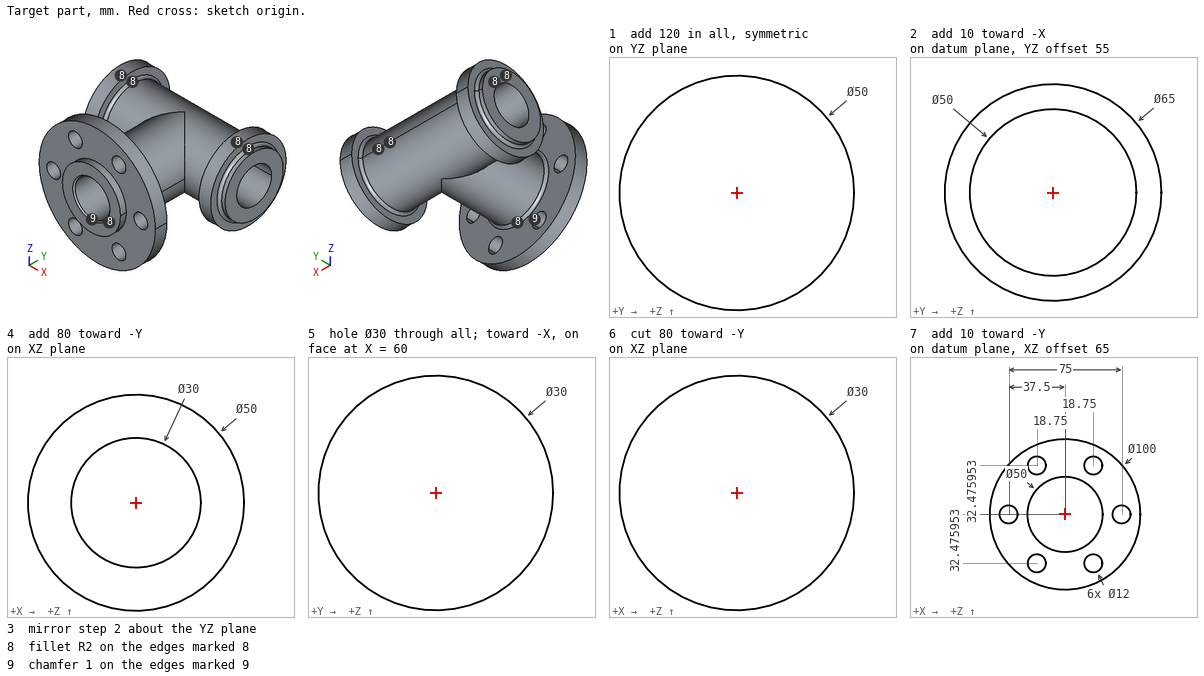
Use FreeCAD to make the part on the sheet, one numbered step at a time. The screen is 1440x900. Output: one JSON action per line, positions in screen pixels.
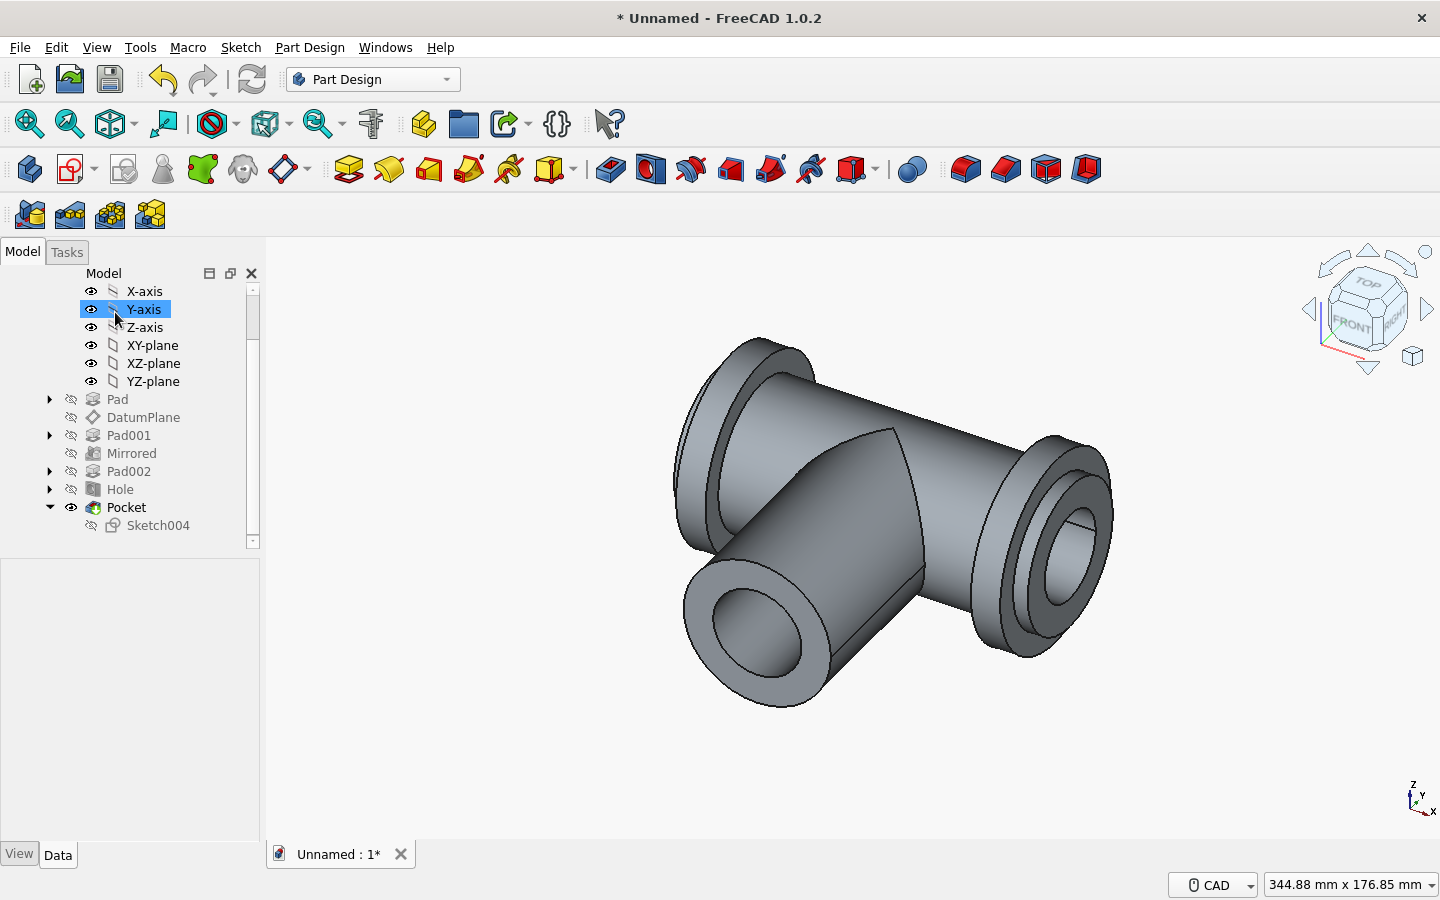
{"action": "scroll", "coordinate": [160, 413], "scroll_direction": "down", "scroll_amount": 3}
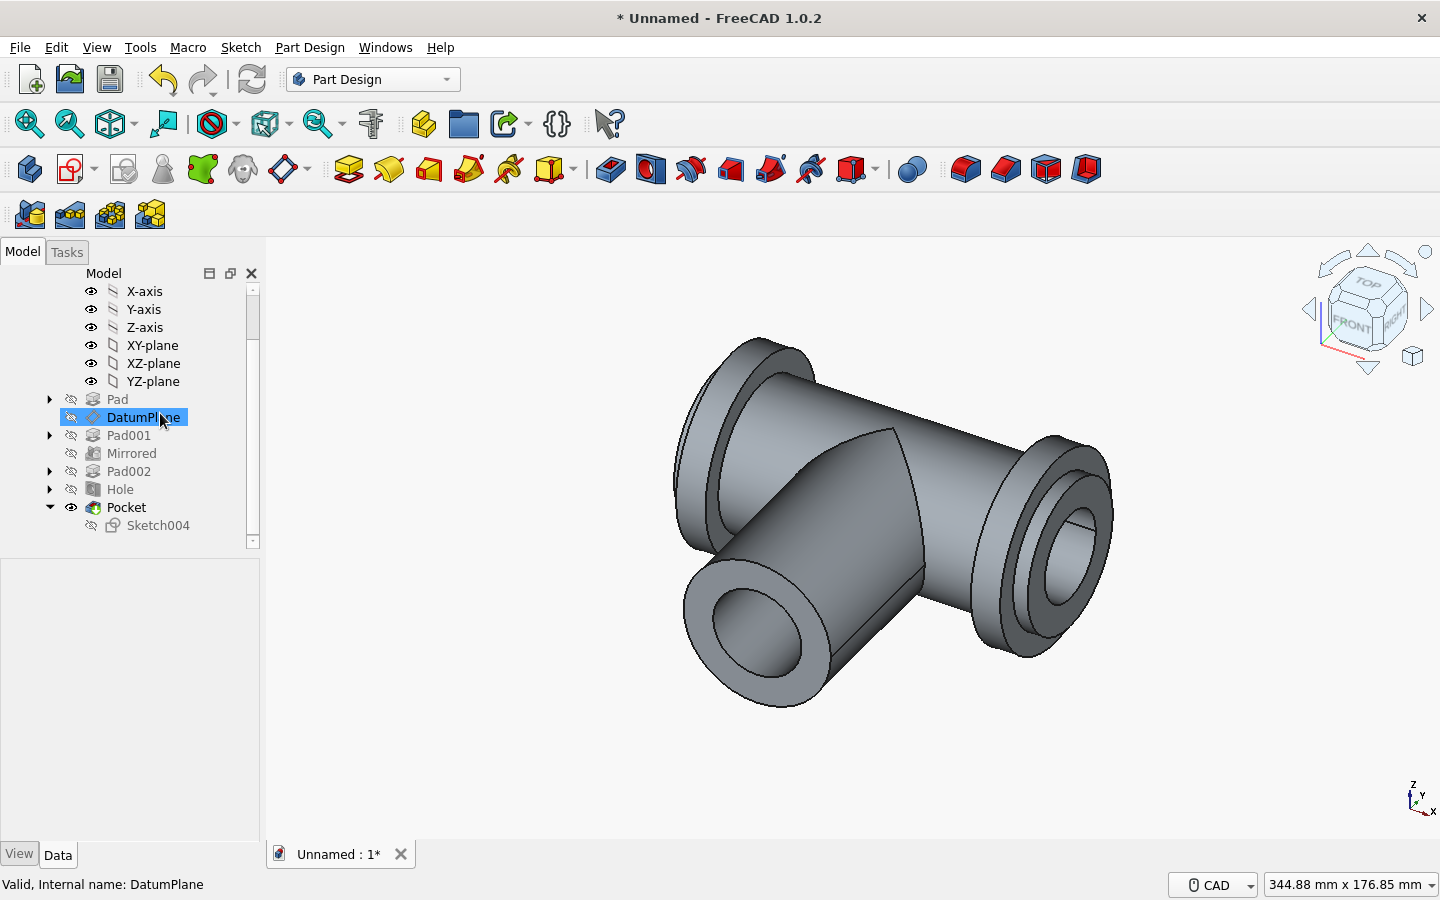
{"action": "scroll", "coordinate": [160, 413], "scroll_direction": "up", "scroll_amount": 15}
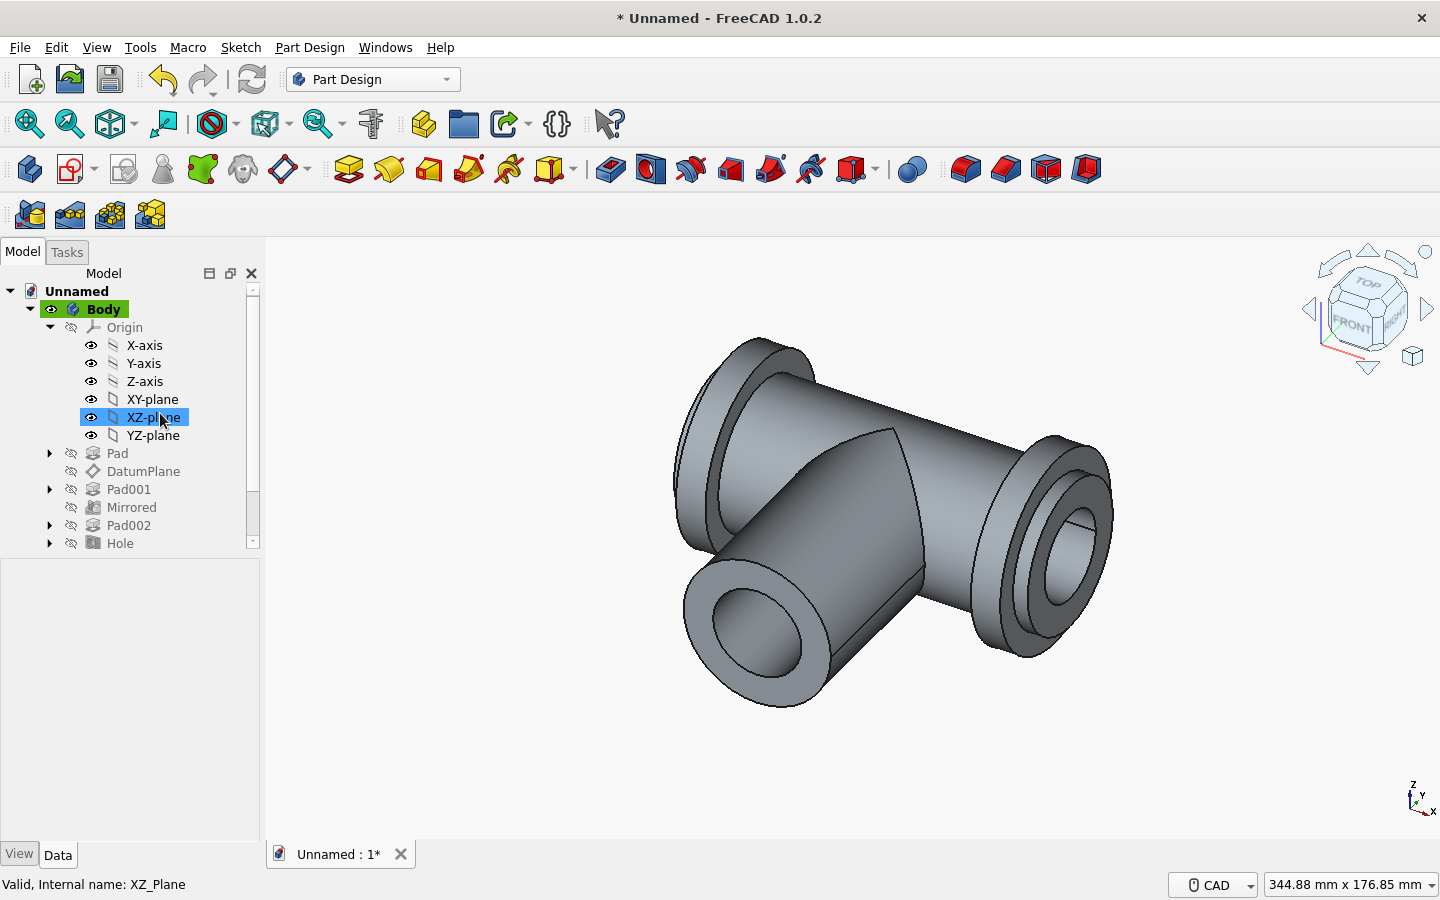
{"action": "left_click", "coordinate": [136, 417]}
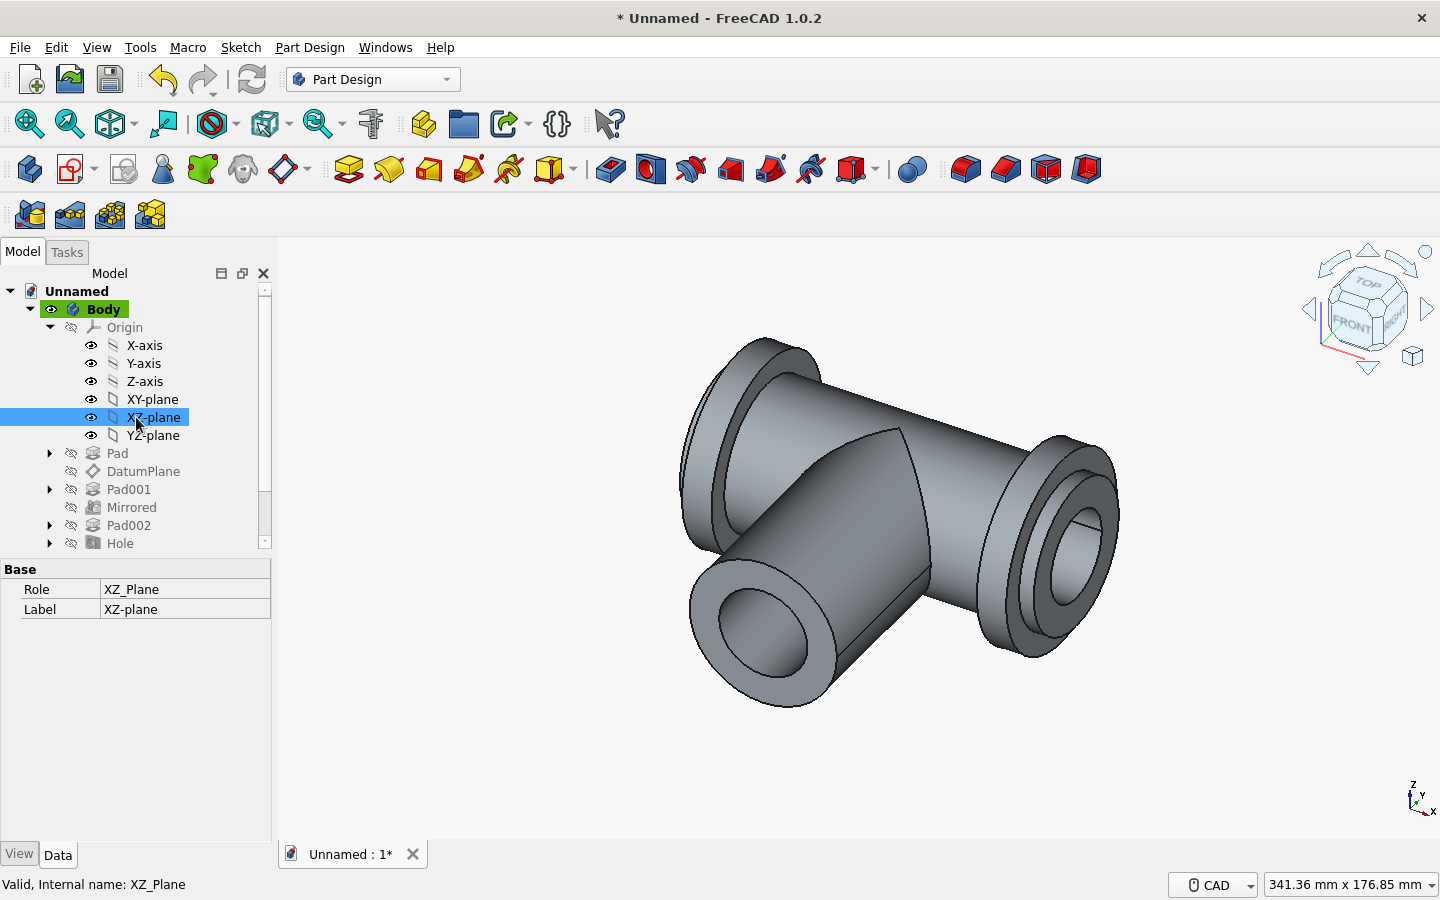
{"action": "left_click", "coordinate": [284, 170]}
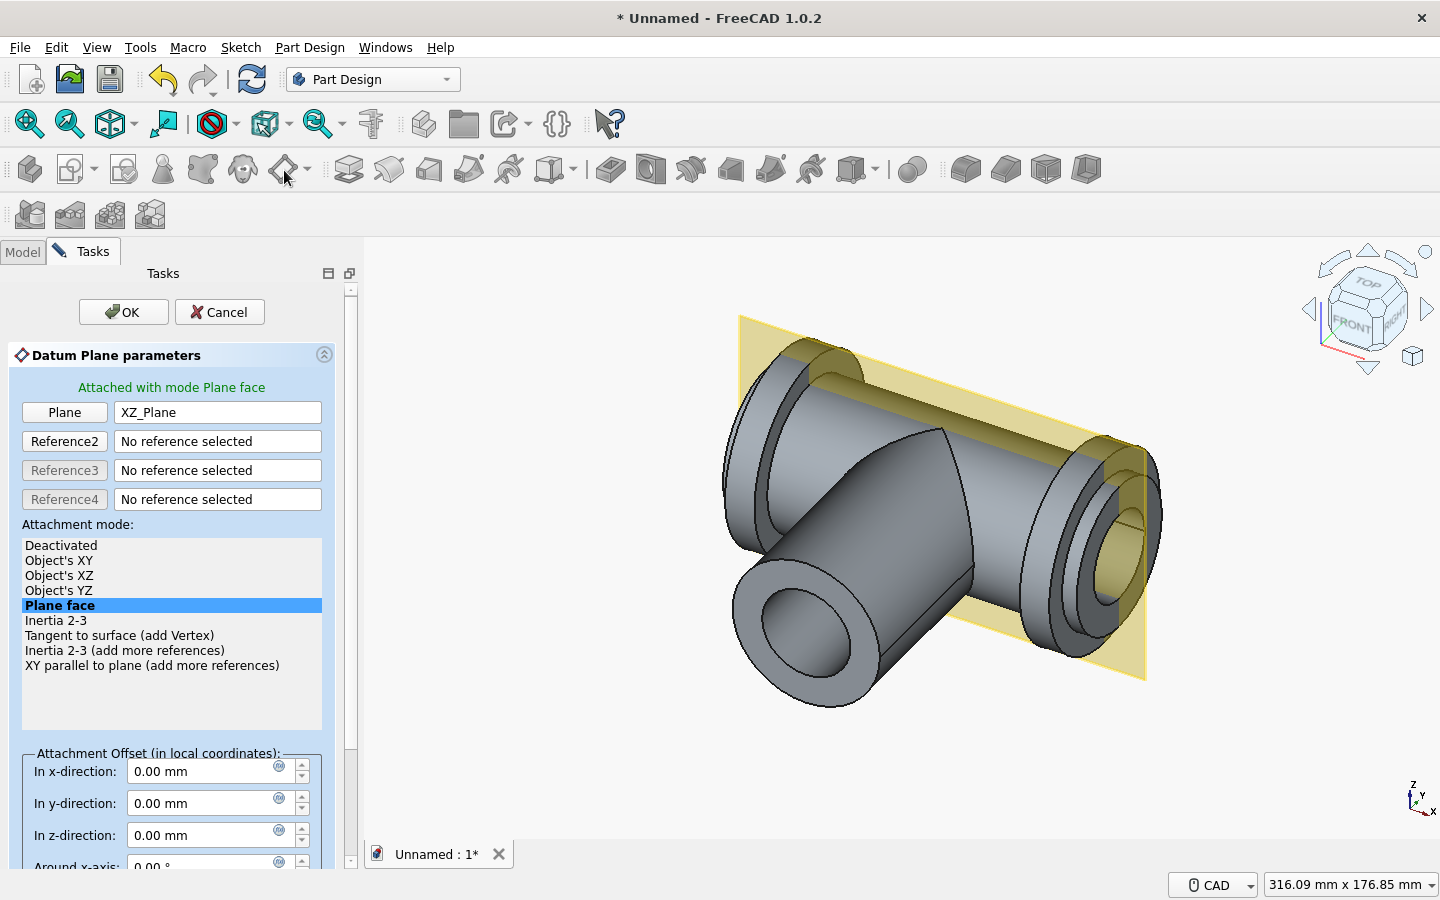
{"action": "triple_click", "coordinate": [210, 835]}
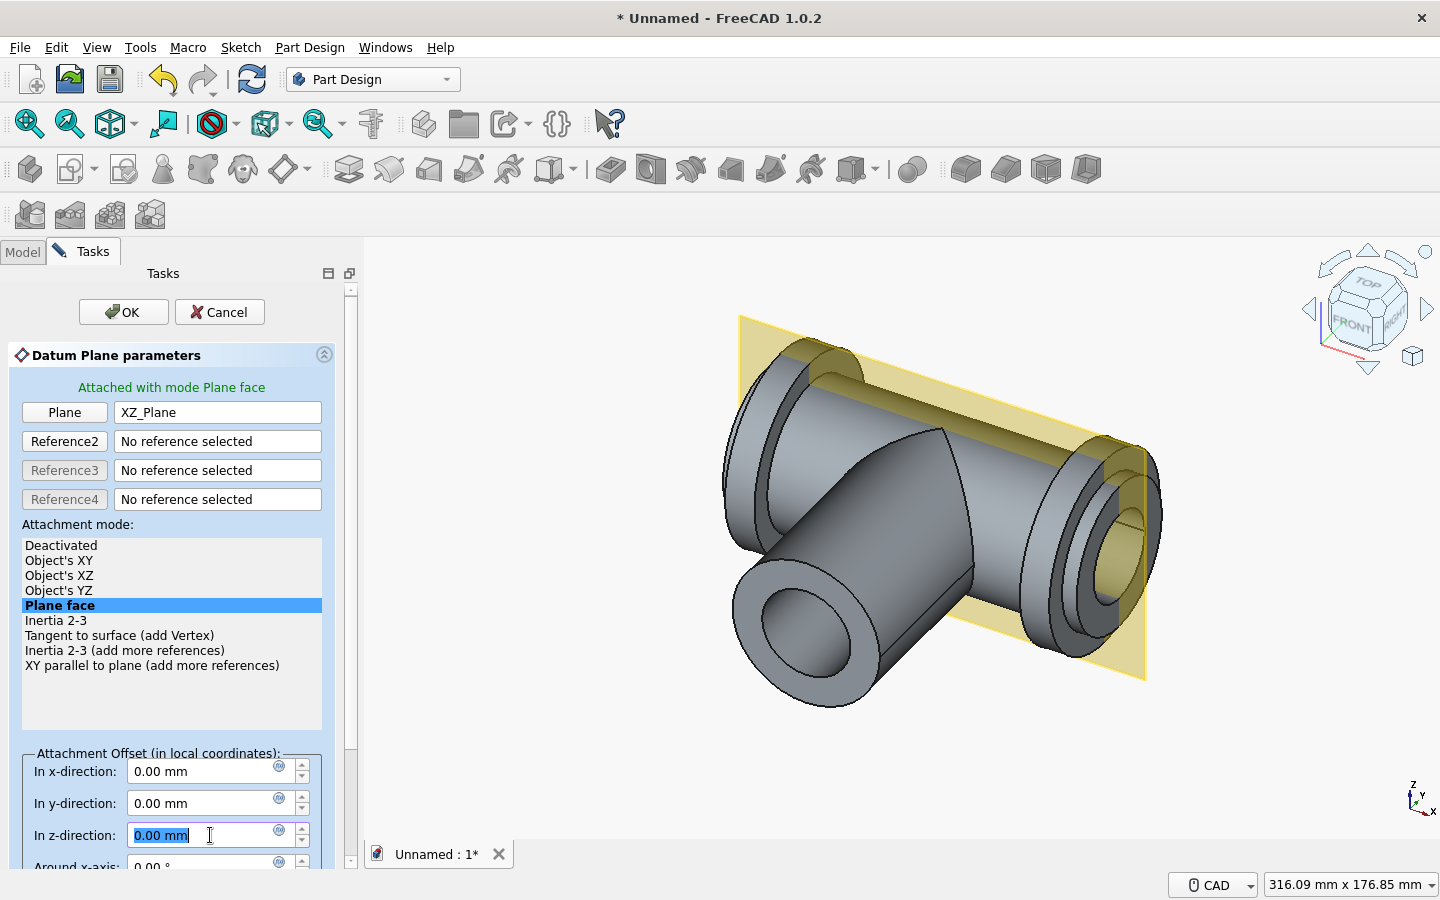
{"action": "type", "text": "65"}
{"action": "key", "text": "Tab"}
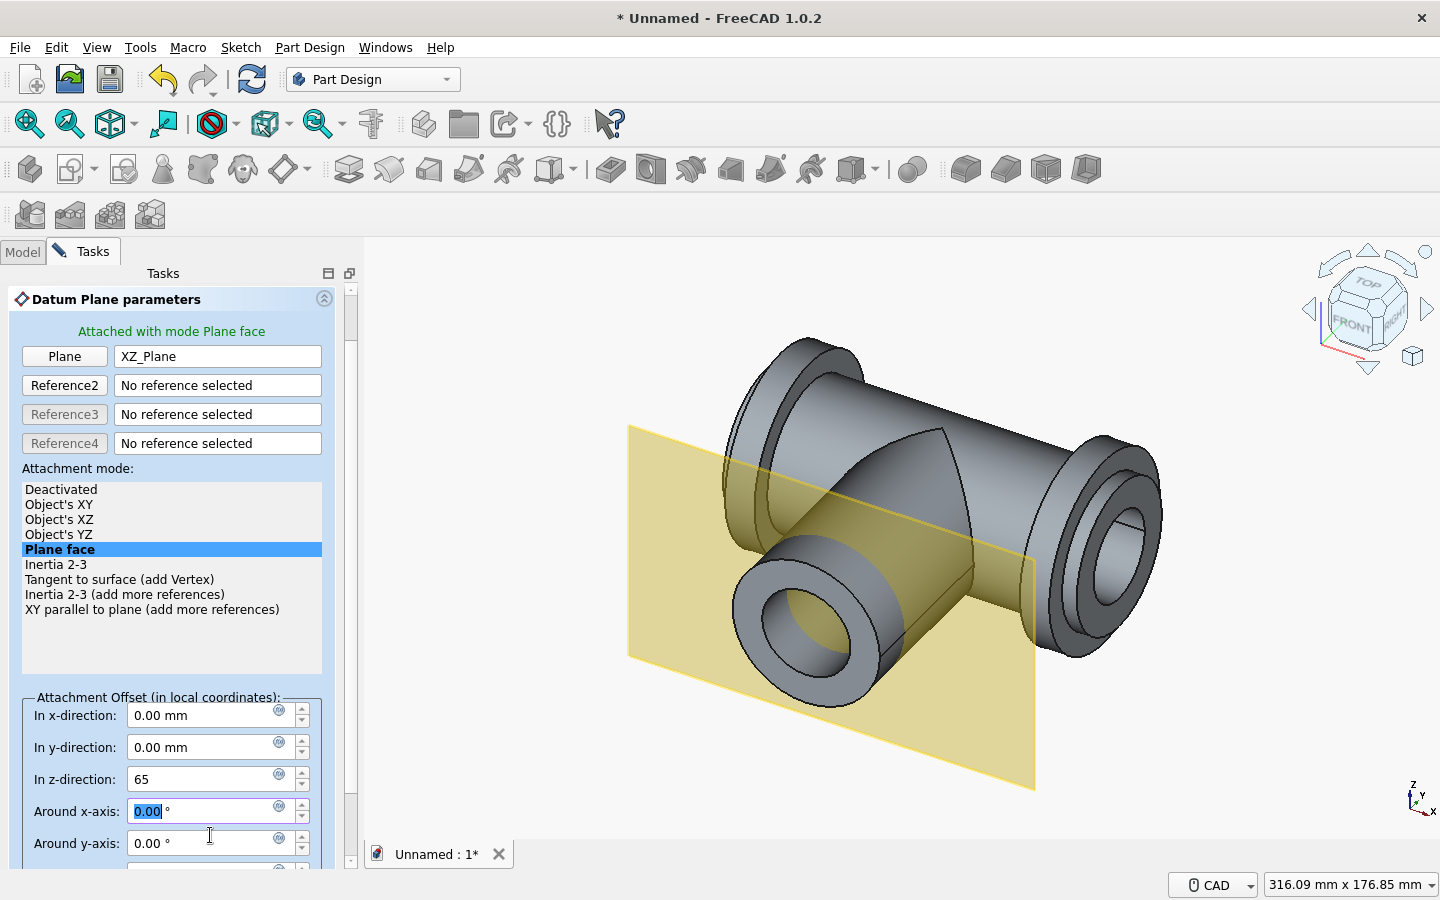
{"action": "scroll", "coordinate": [351, 576], "scroll_direction": "up", "scroll_amount": 2}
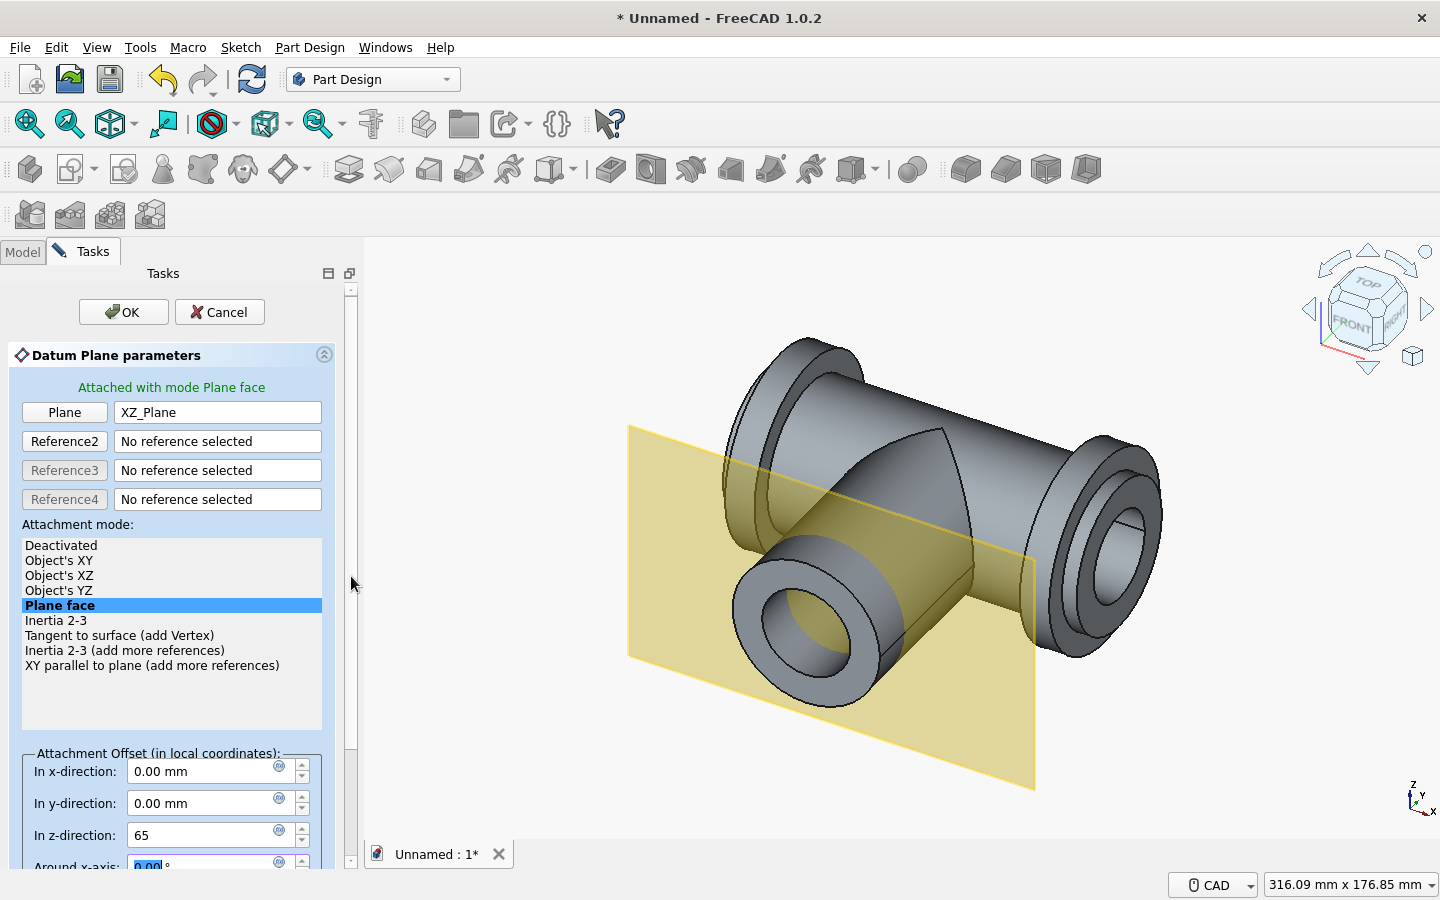
{"action": "left_click", "coordinate": [124, 312]}